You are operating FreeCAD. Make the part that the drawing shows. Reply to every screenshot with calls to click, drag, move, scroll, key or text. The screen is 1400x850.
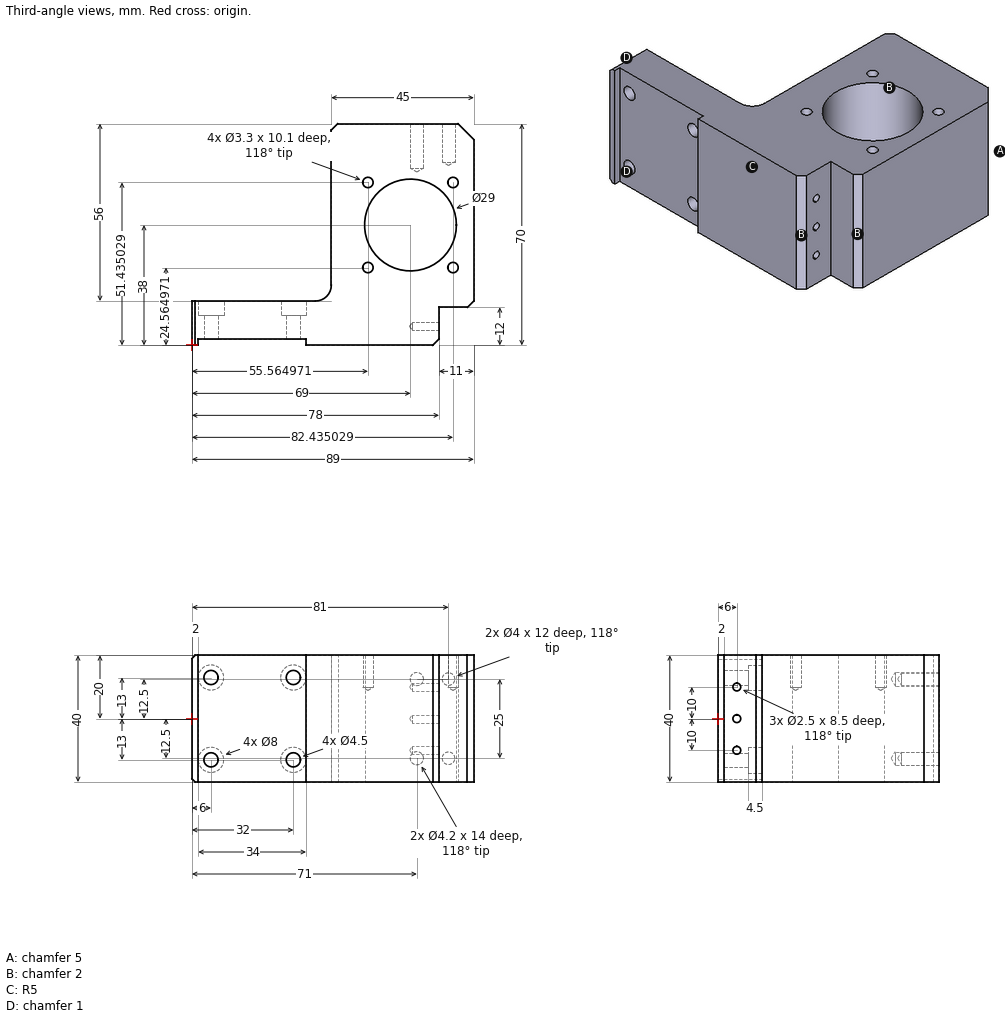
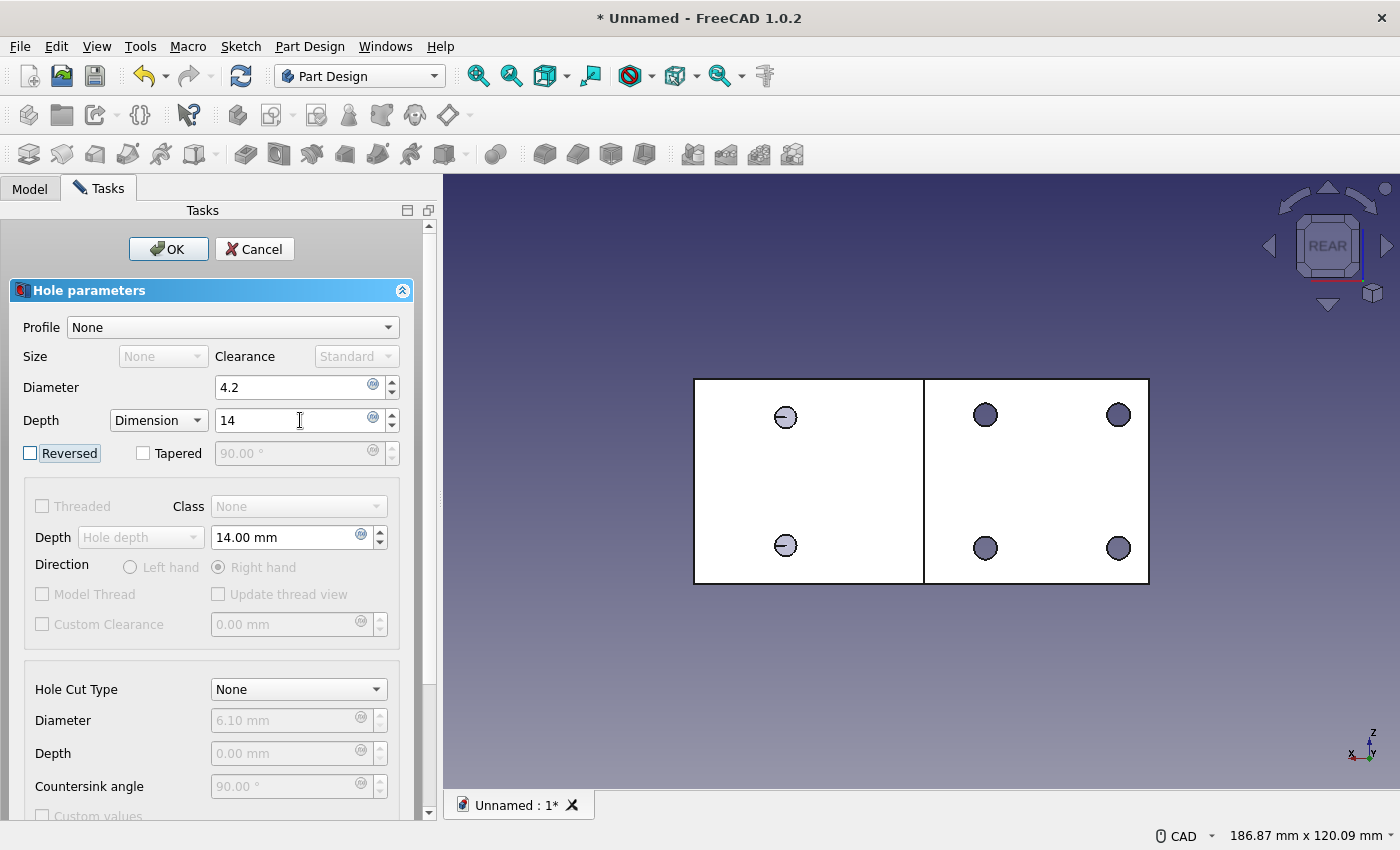
click(169, 249)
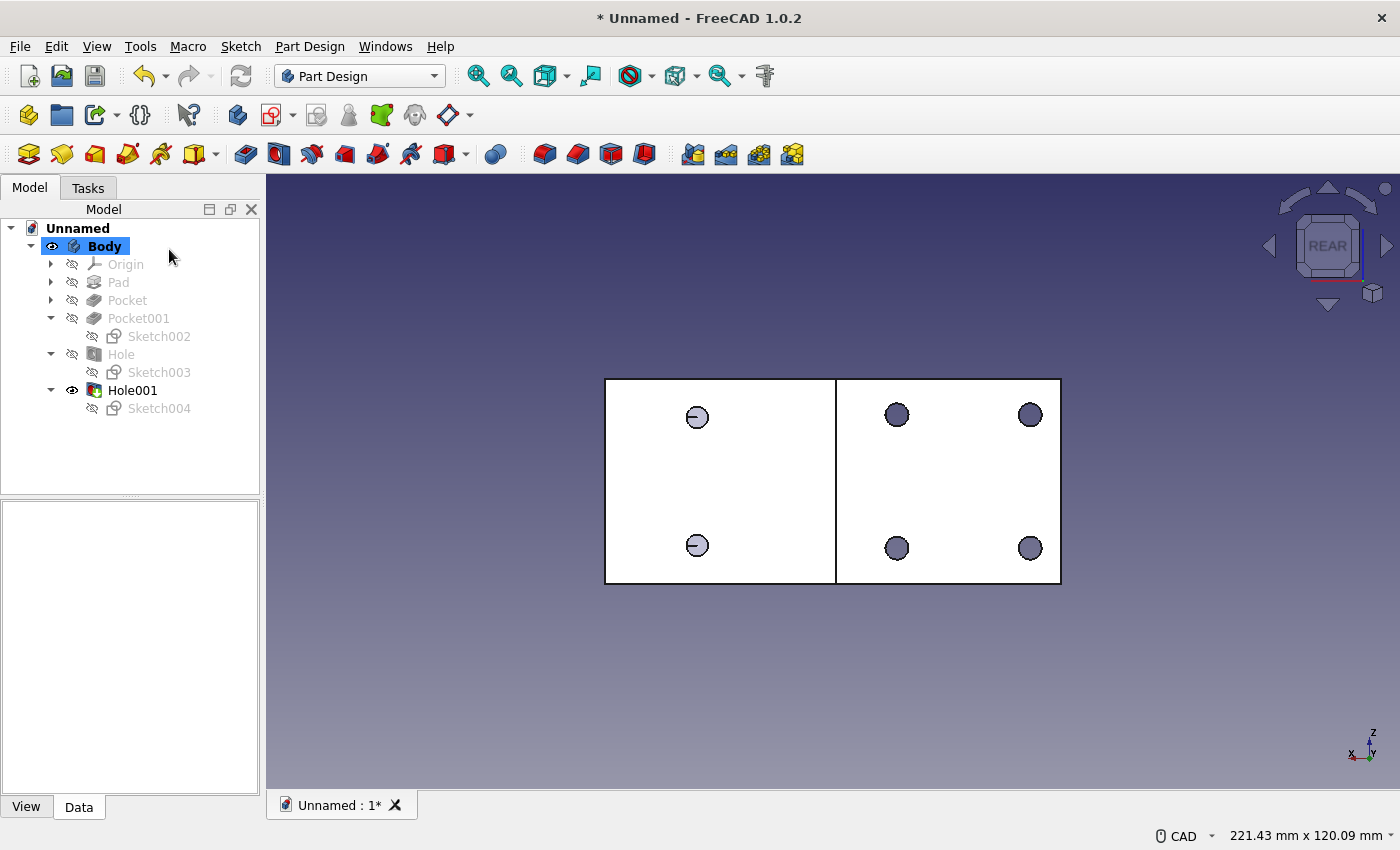
click(479, 76)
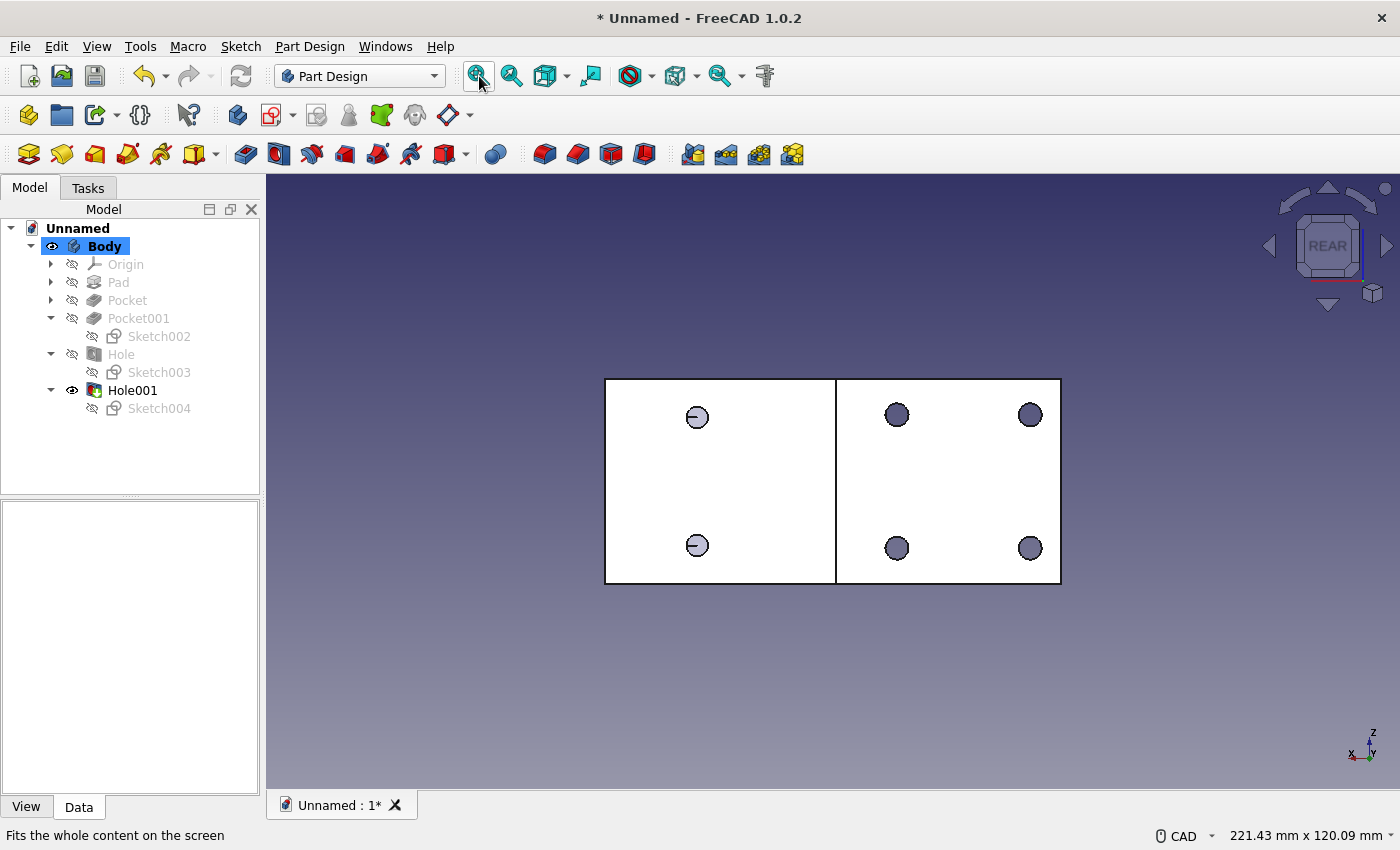
click(753, 480)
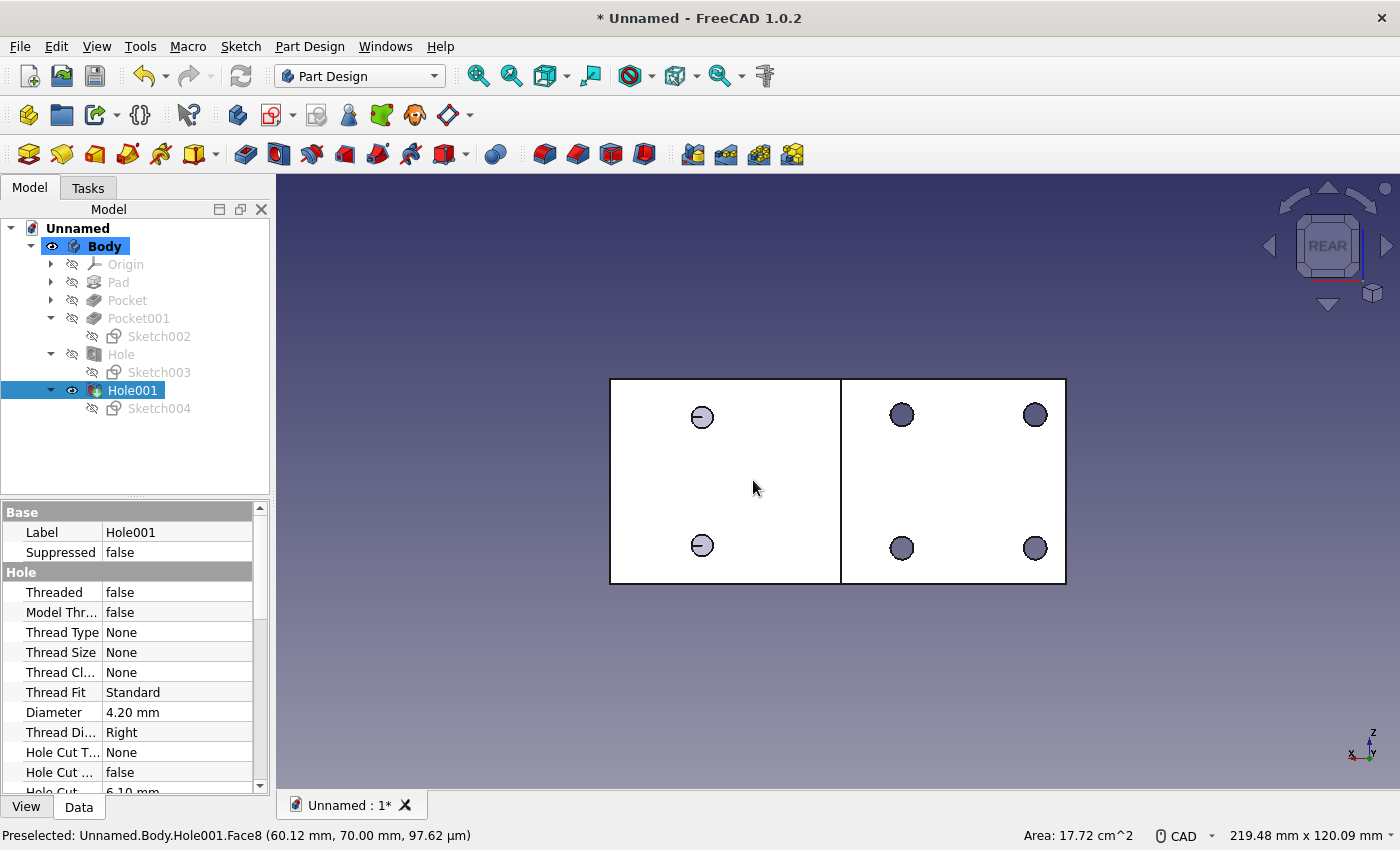
click(270, 116)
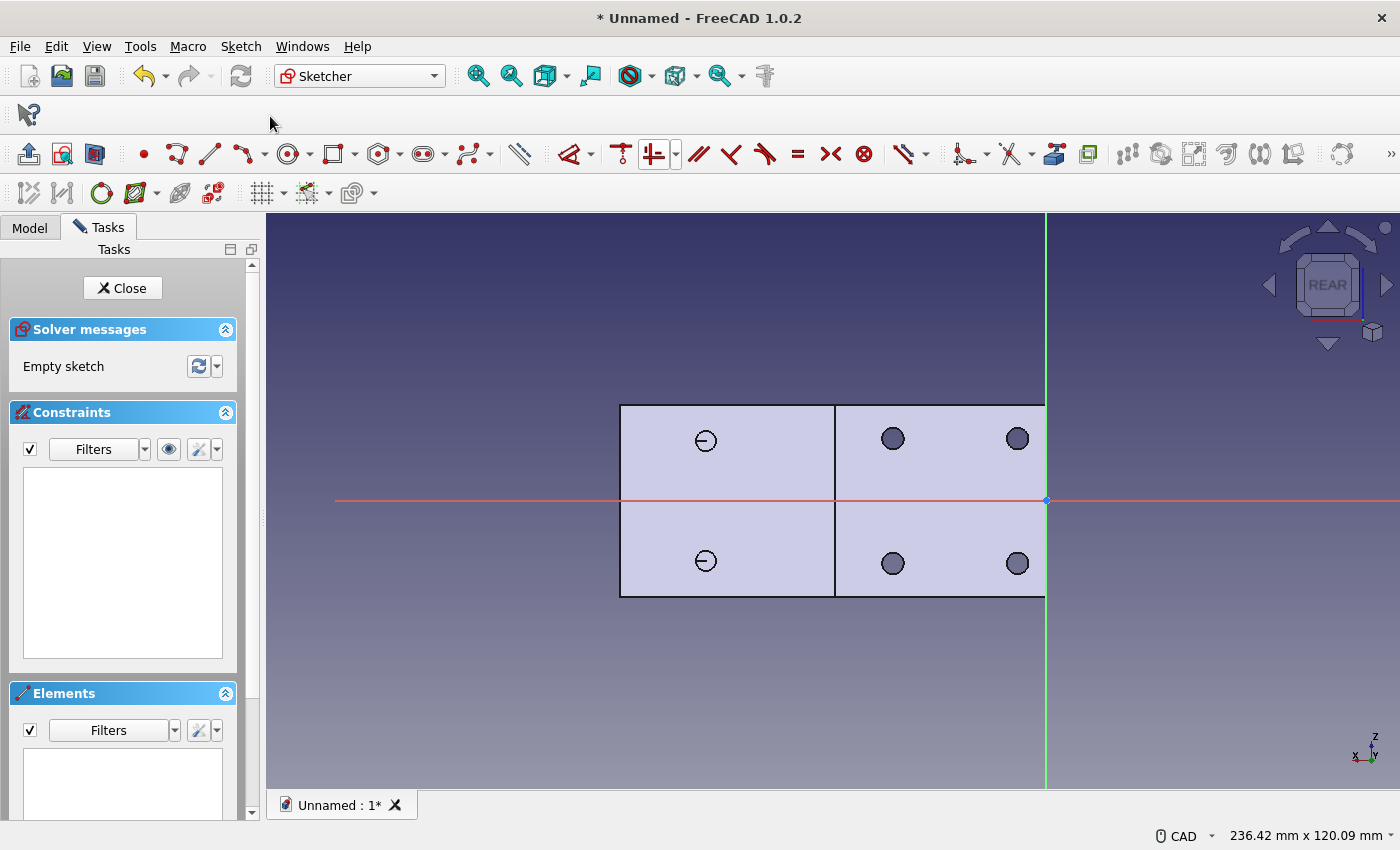
scroll(596, 501, up, 5)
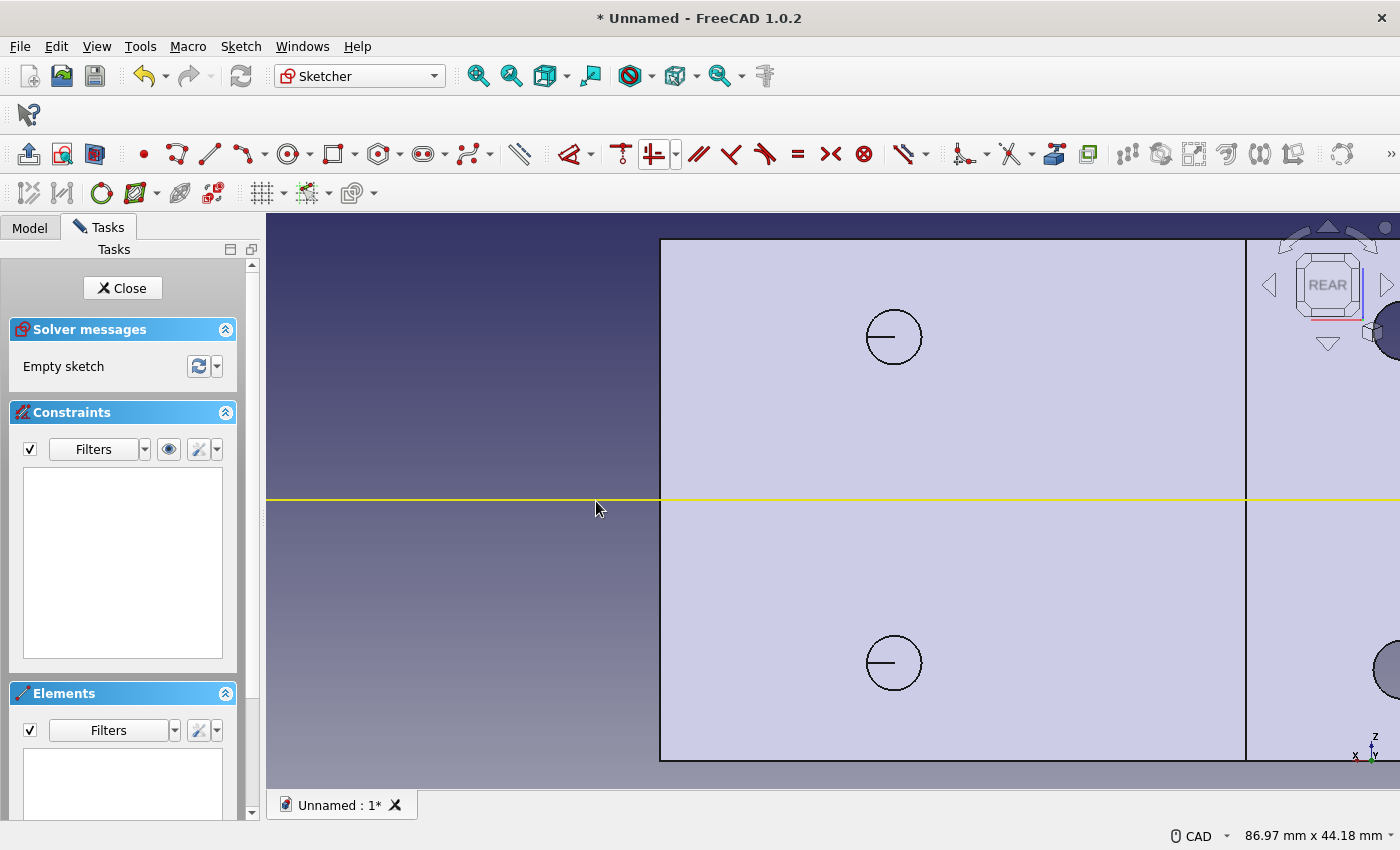
click(288, 154)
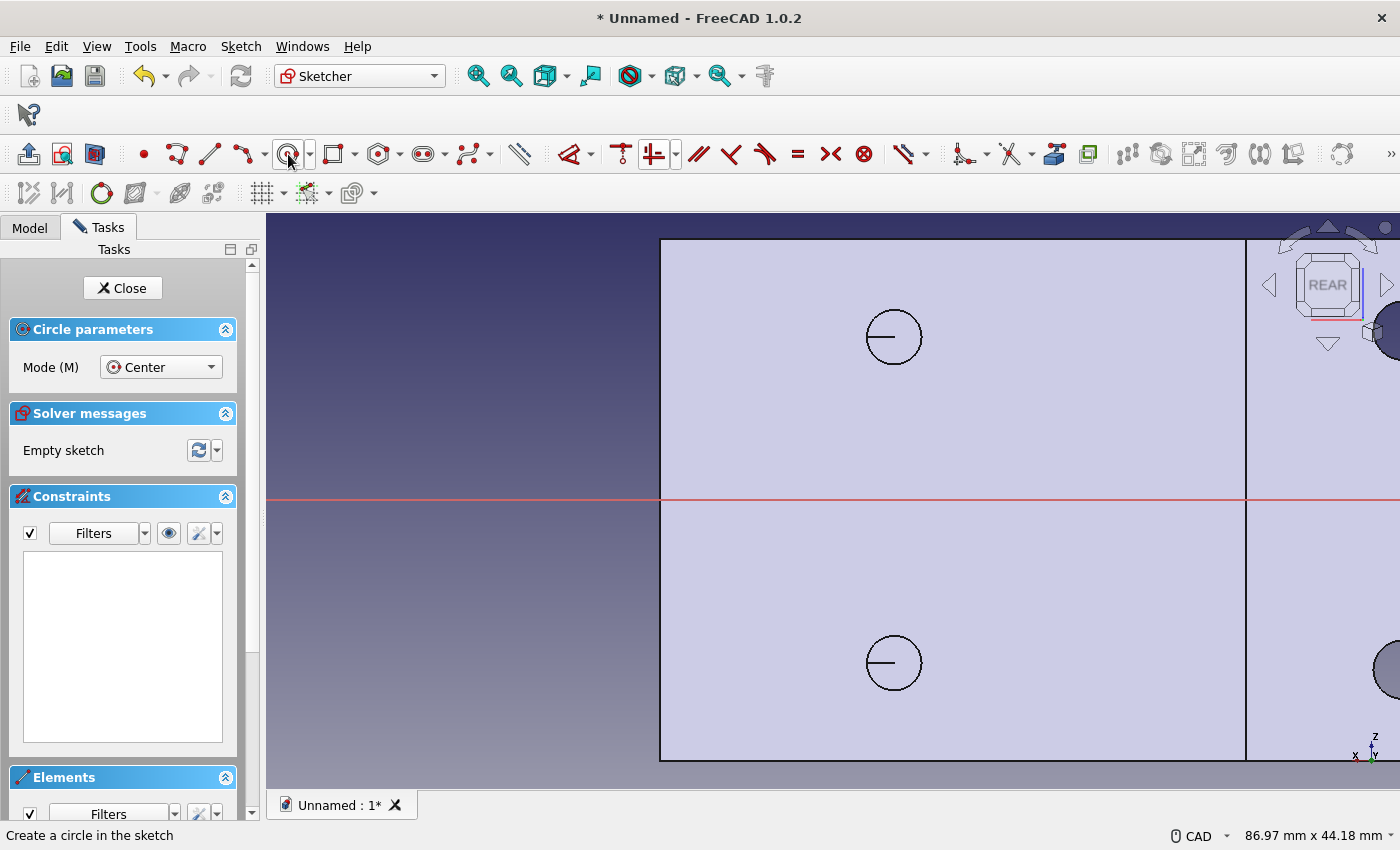
click(764, 337)
move(782, 319)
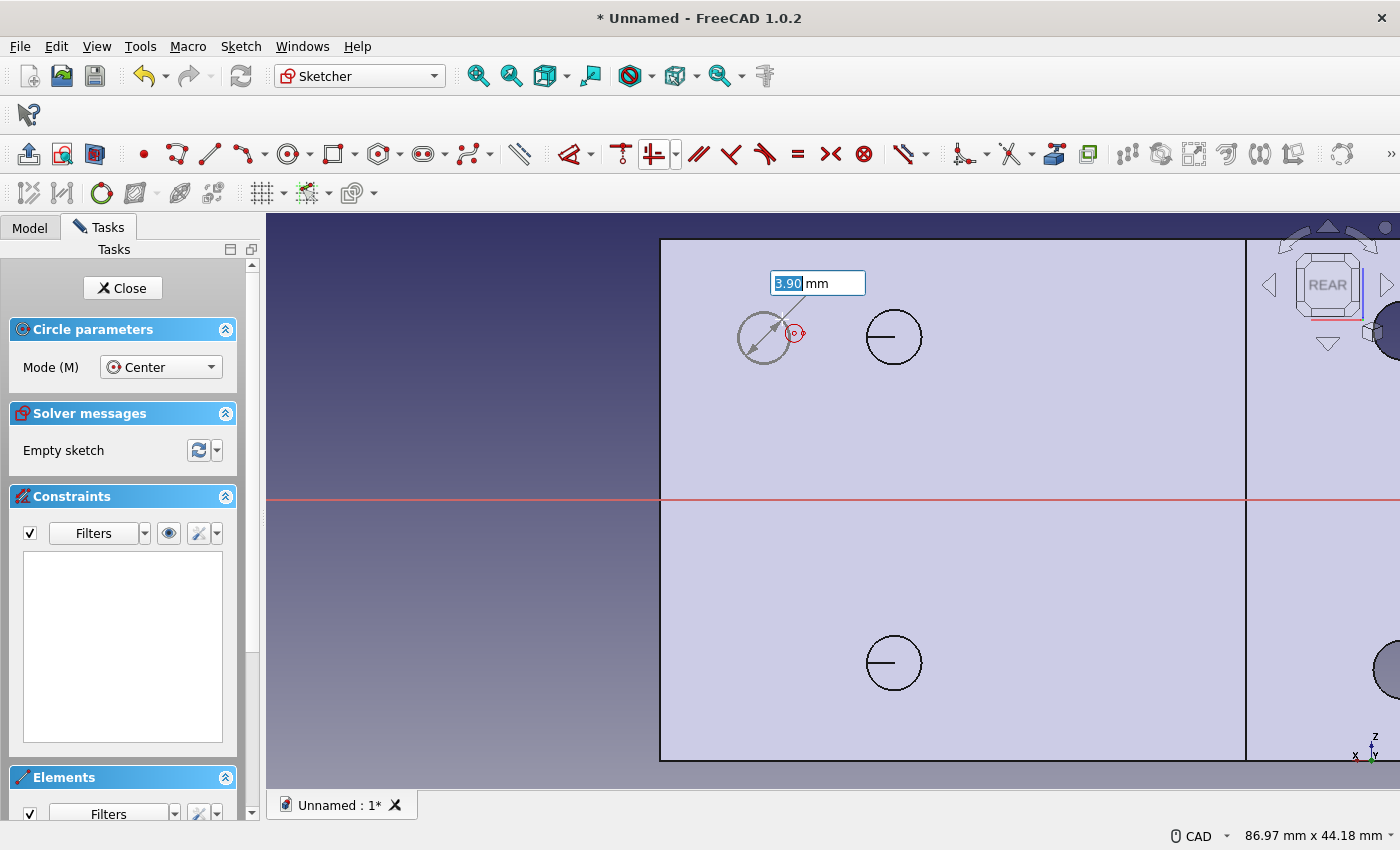
text(4)
key(Return)